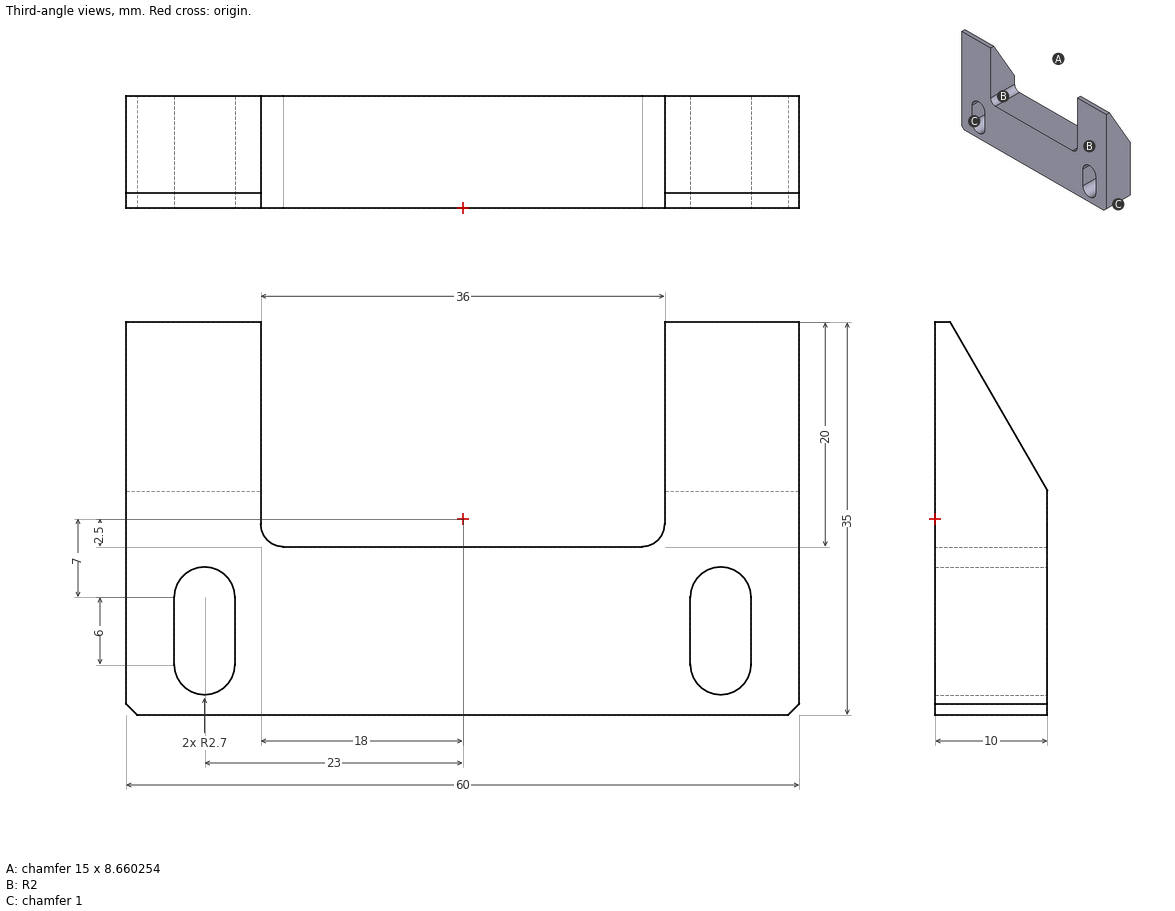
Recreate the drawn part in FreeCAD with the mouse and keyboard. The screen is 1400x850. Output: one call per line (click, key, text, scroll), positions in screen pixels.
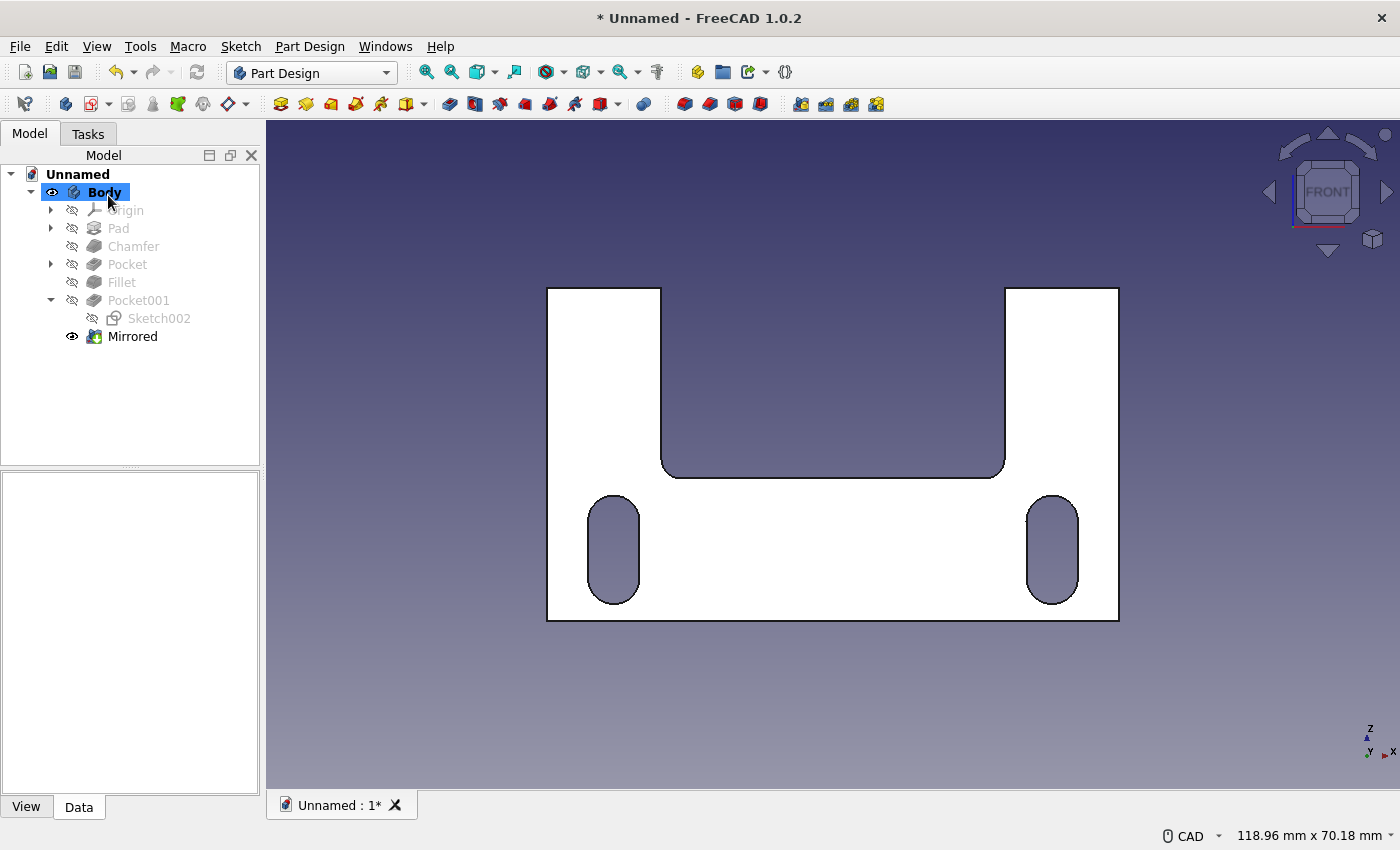
key(3)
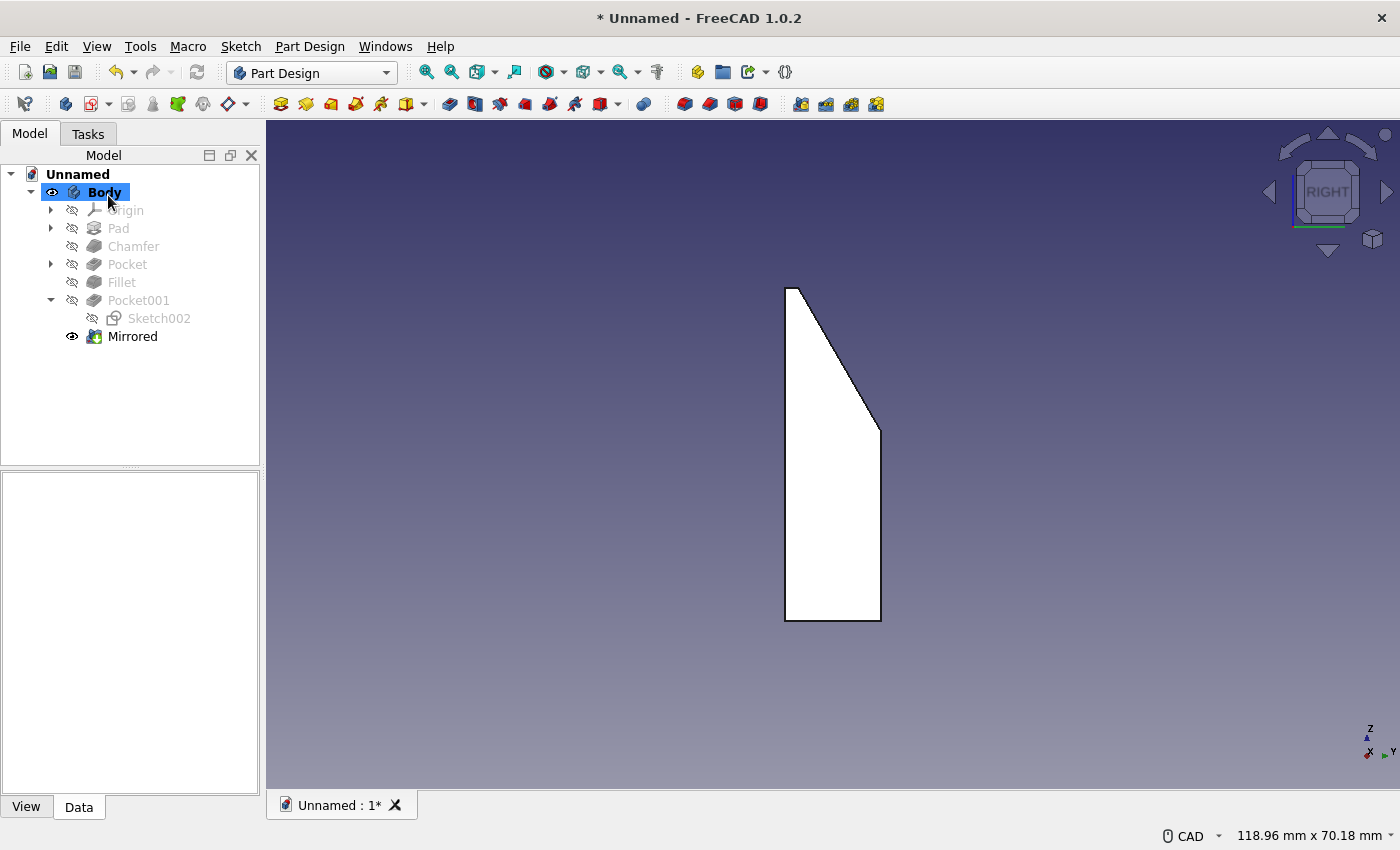
click(833, 620)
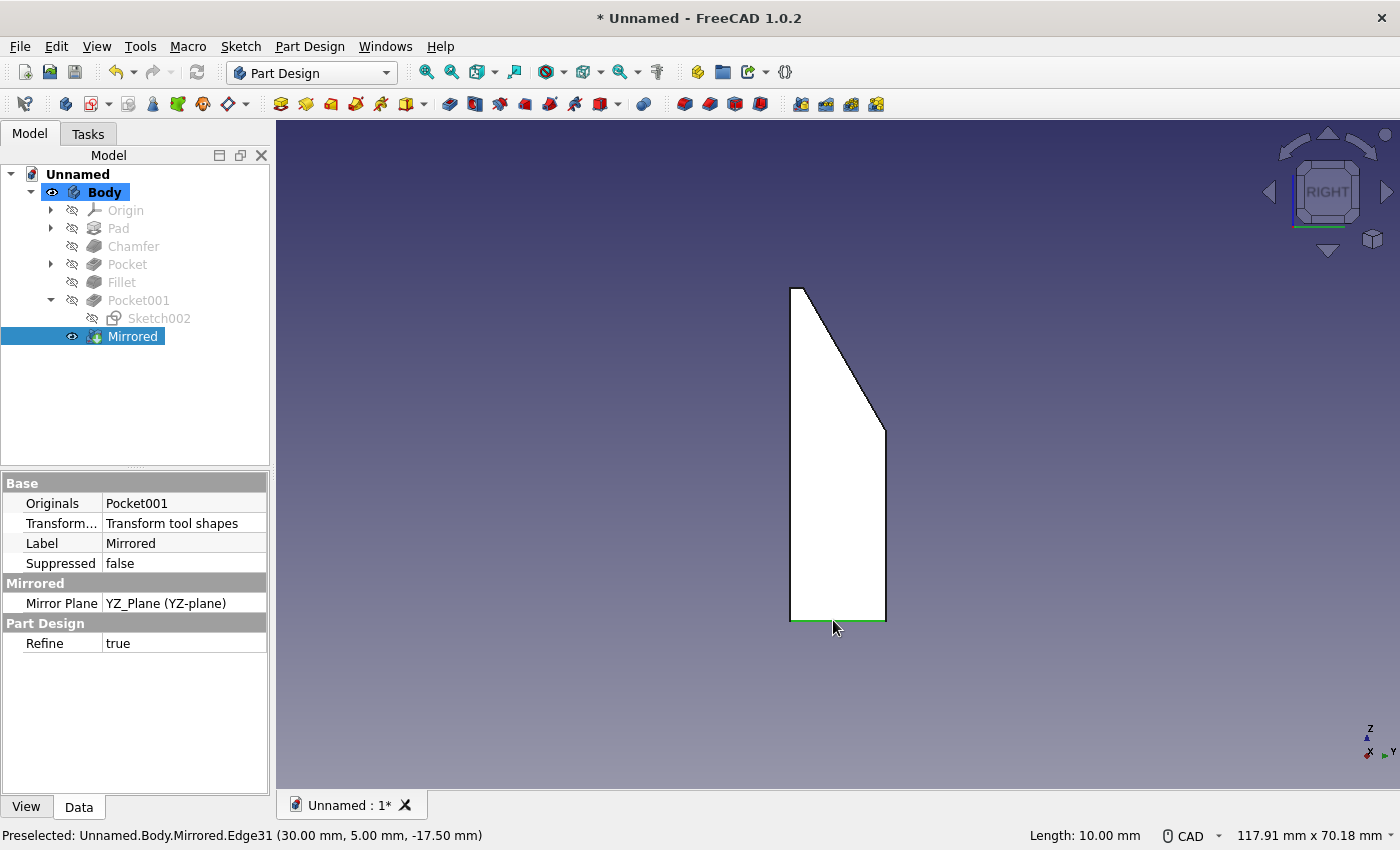
key(5)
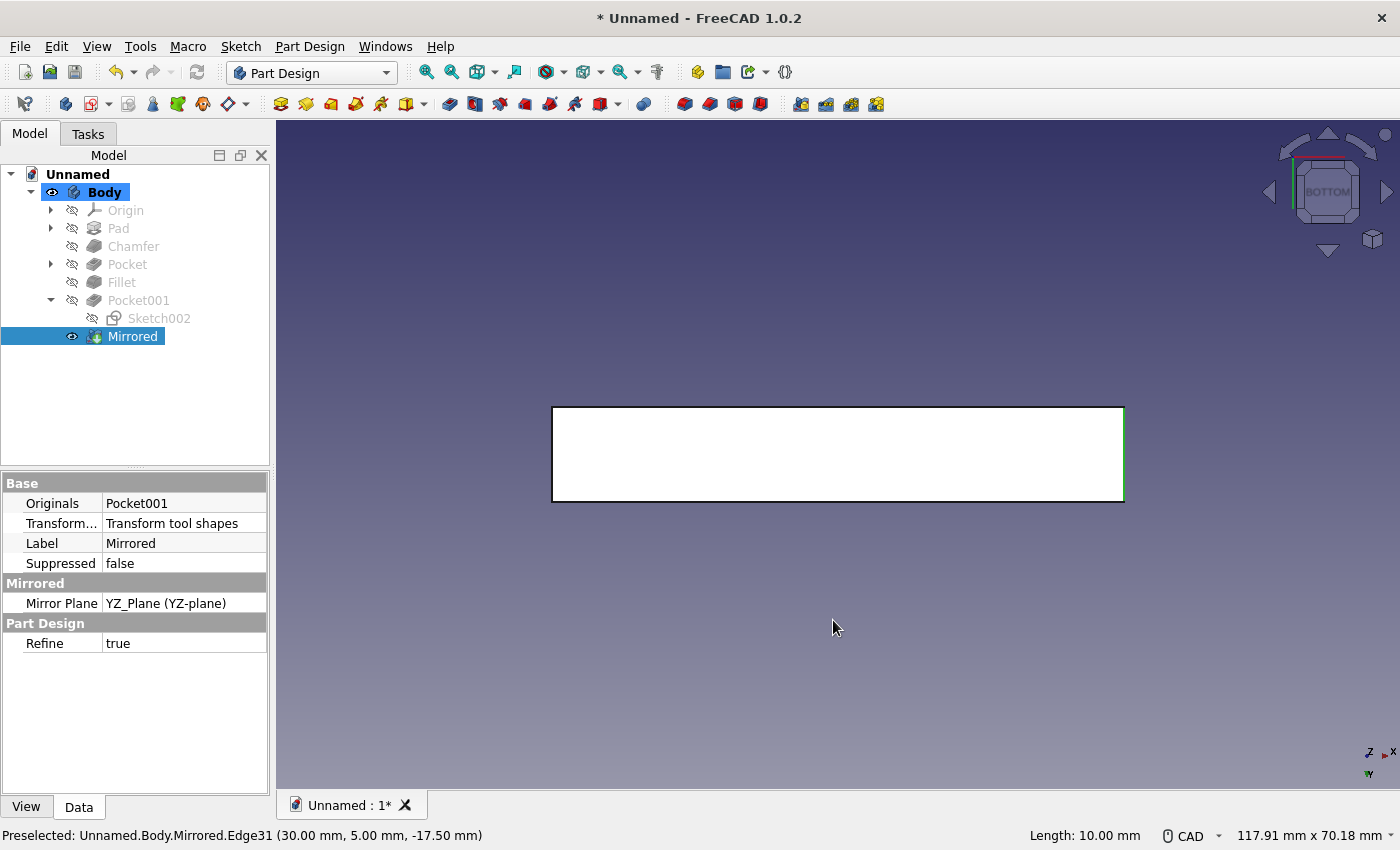
click(552, 454, ctrl)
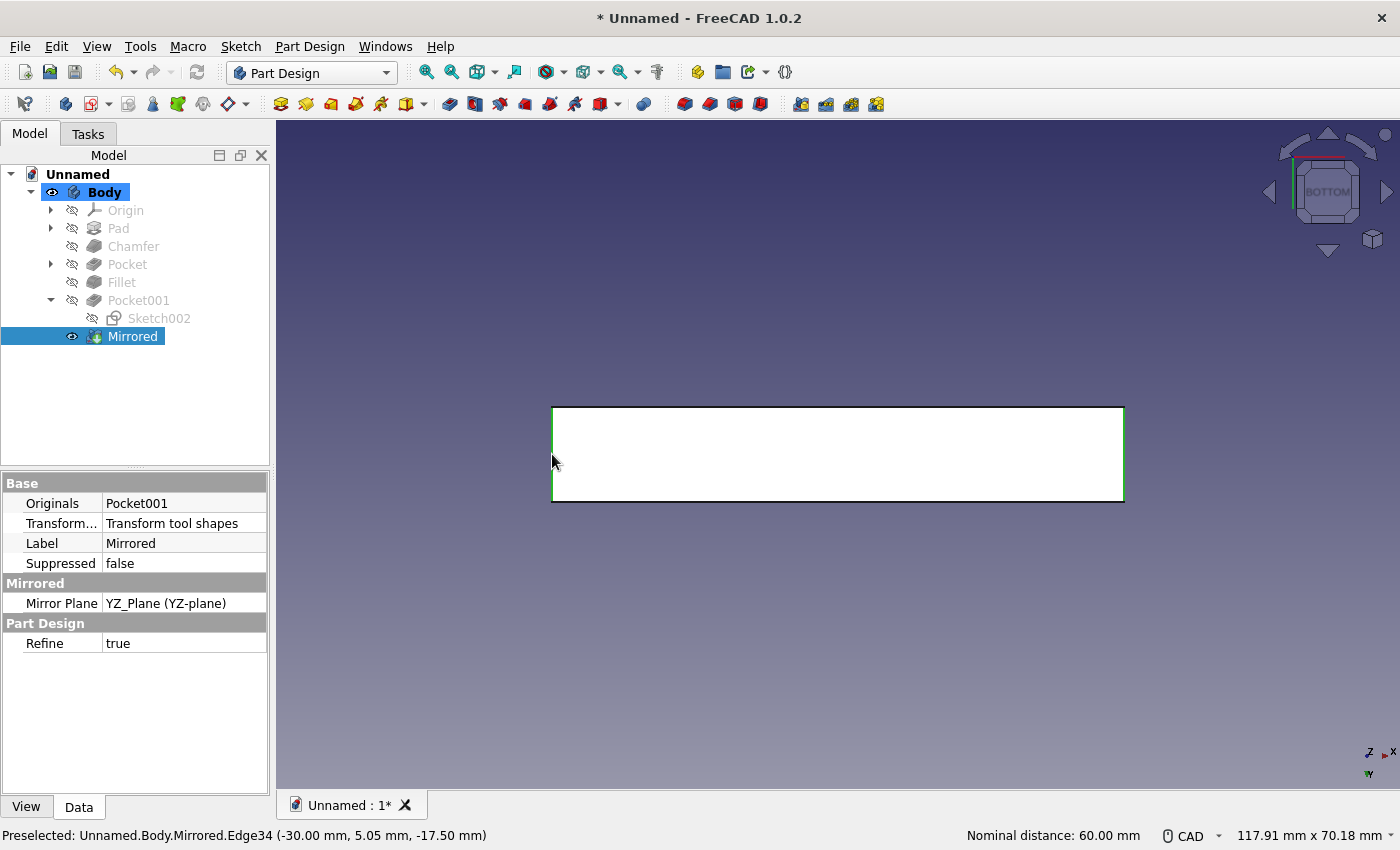
click(710, 104)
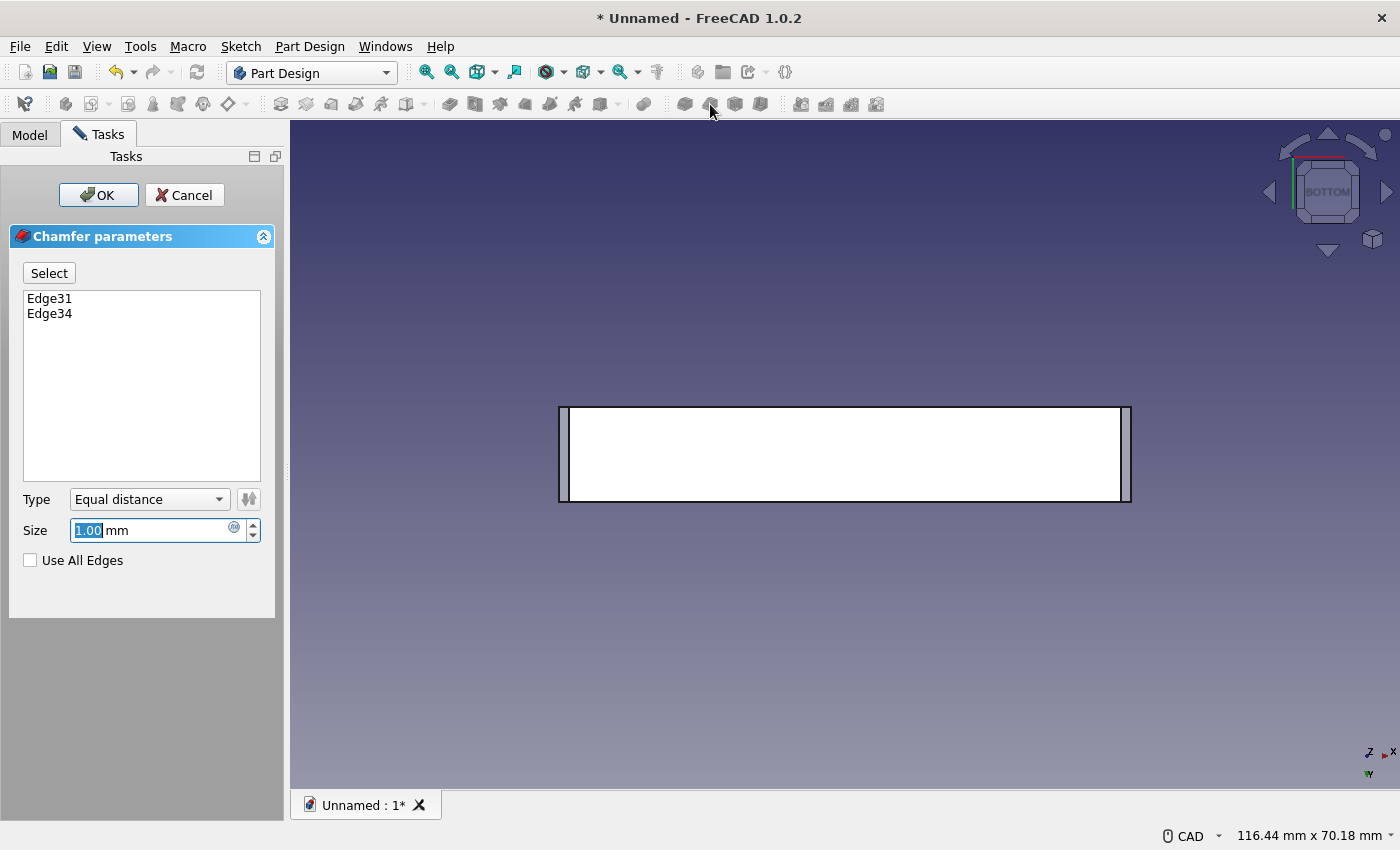
text(1)
key(Tab)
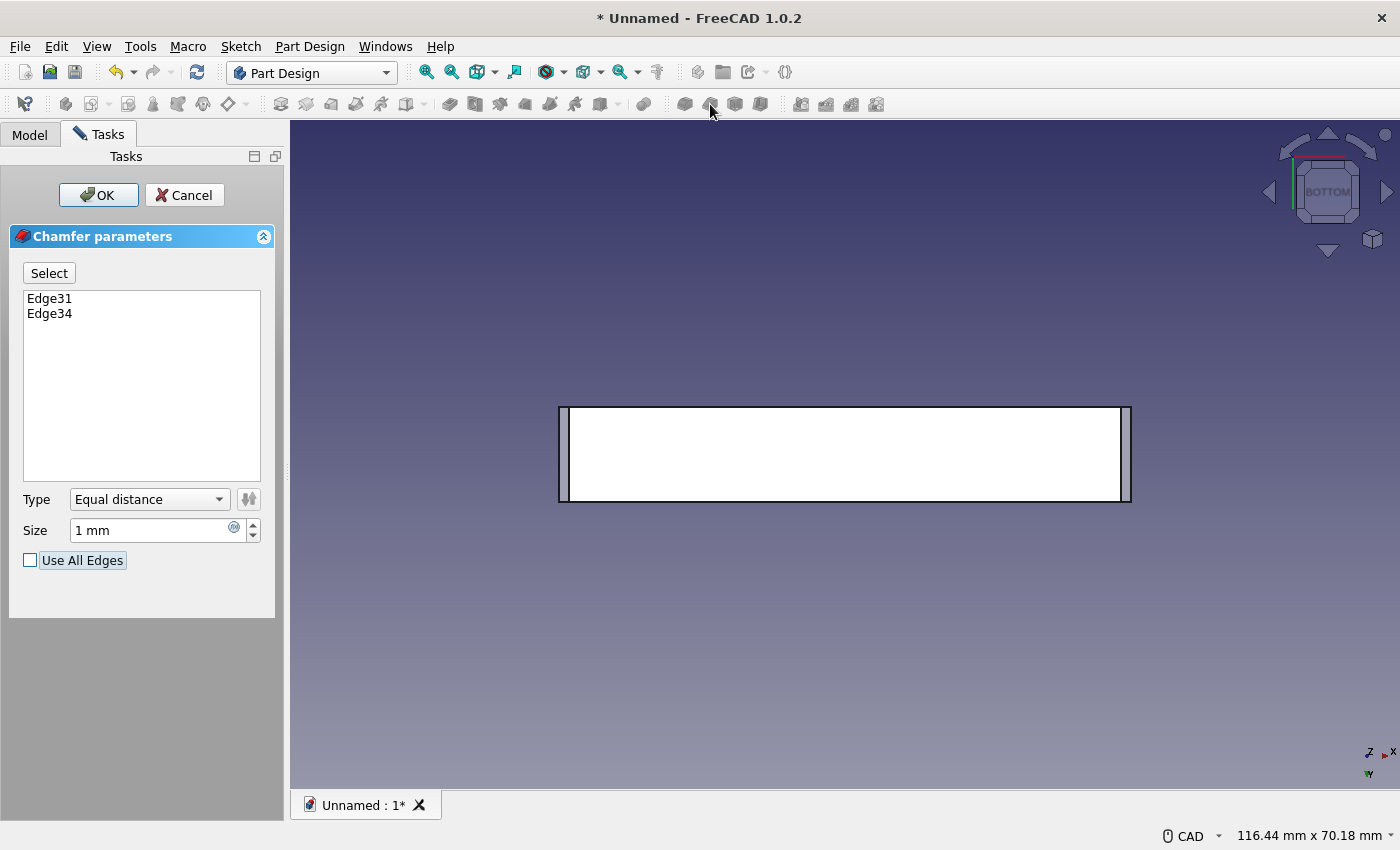
click(99, 195)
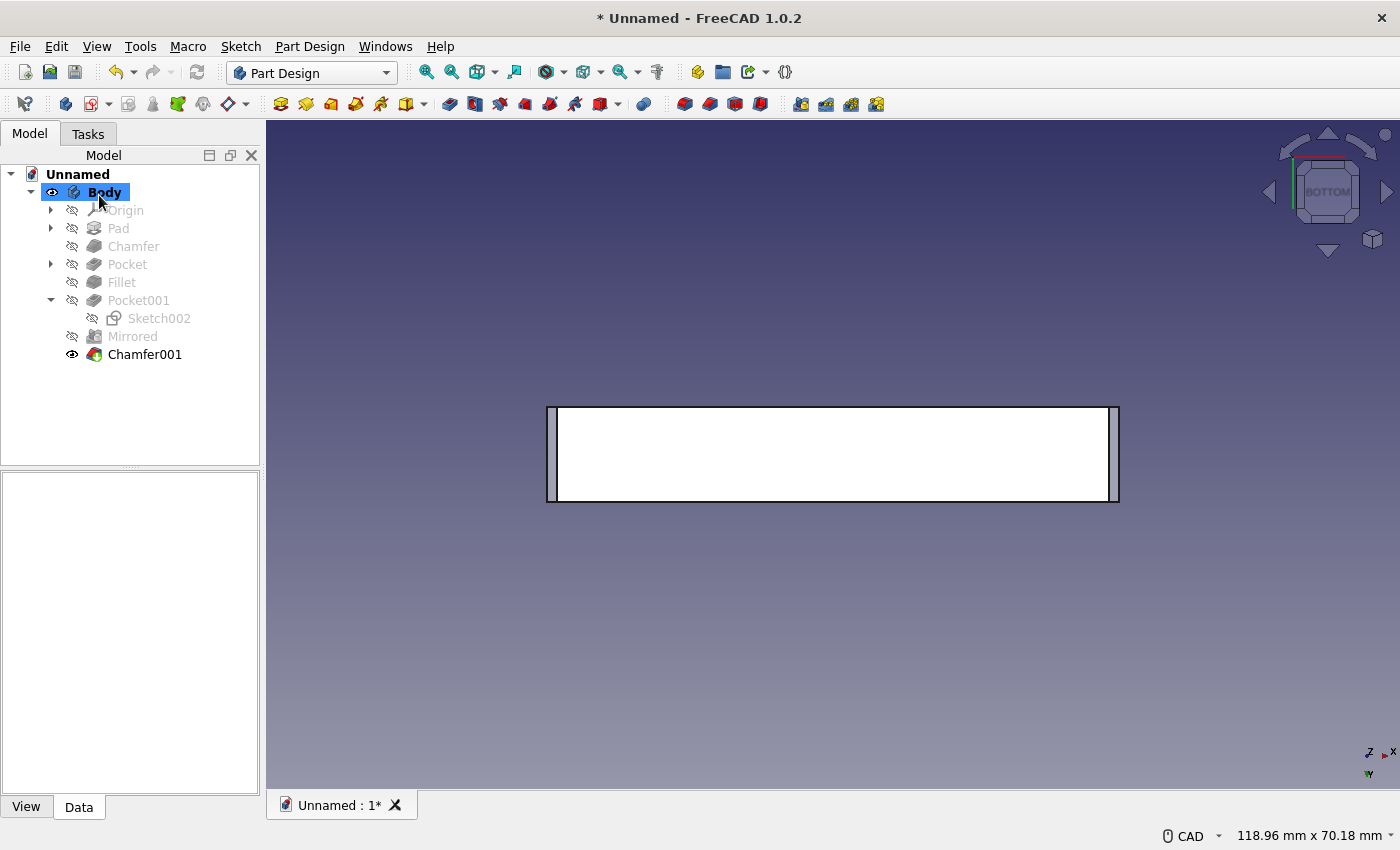
key(0)